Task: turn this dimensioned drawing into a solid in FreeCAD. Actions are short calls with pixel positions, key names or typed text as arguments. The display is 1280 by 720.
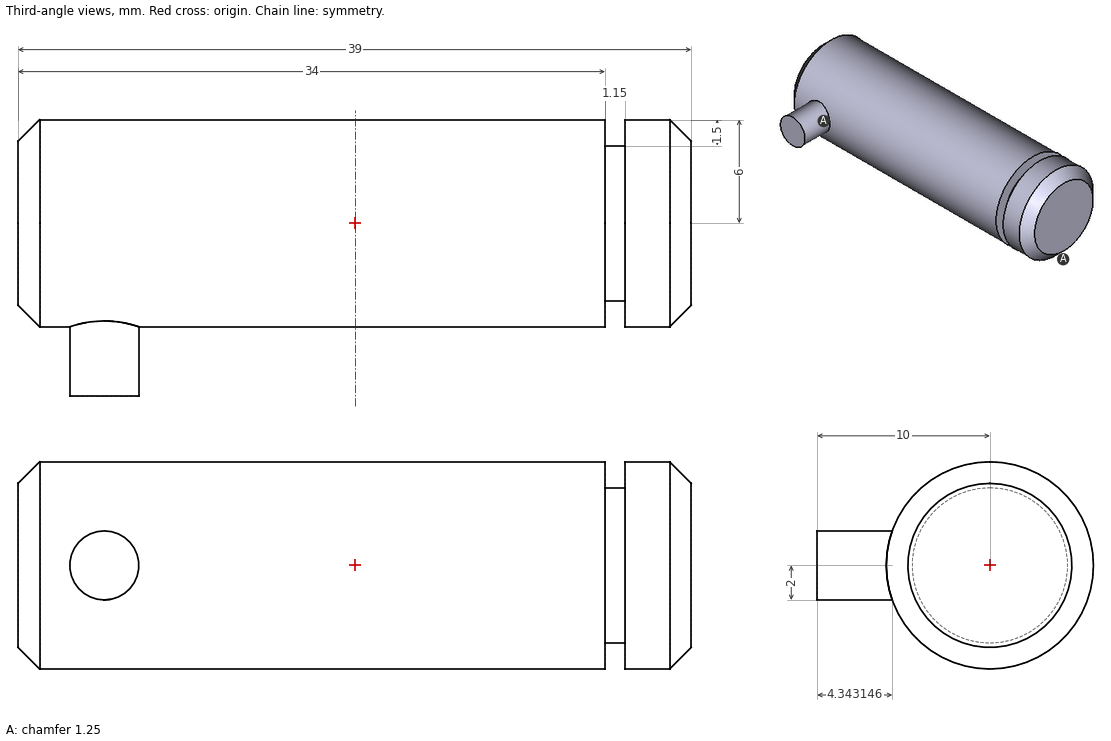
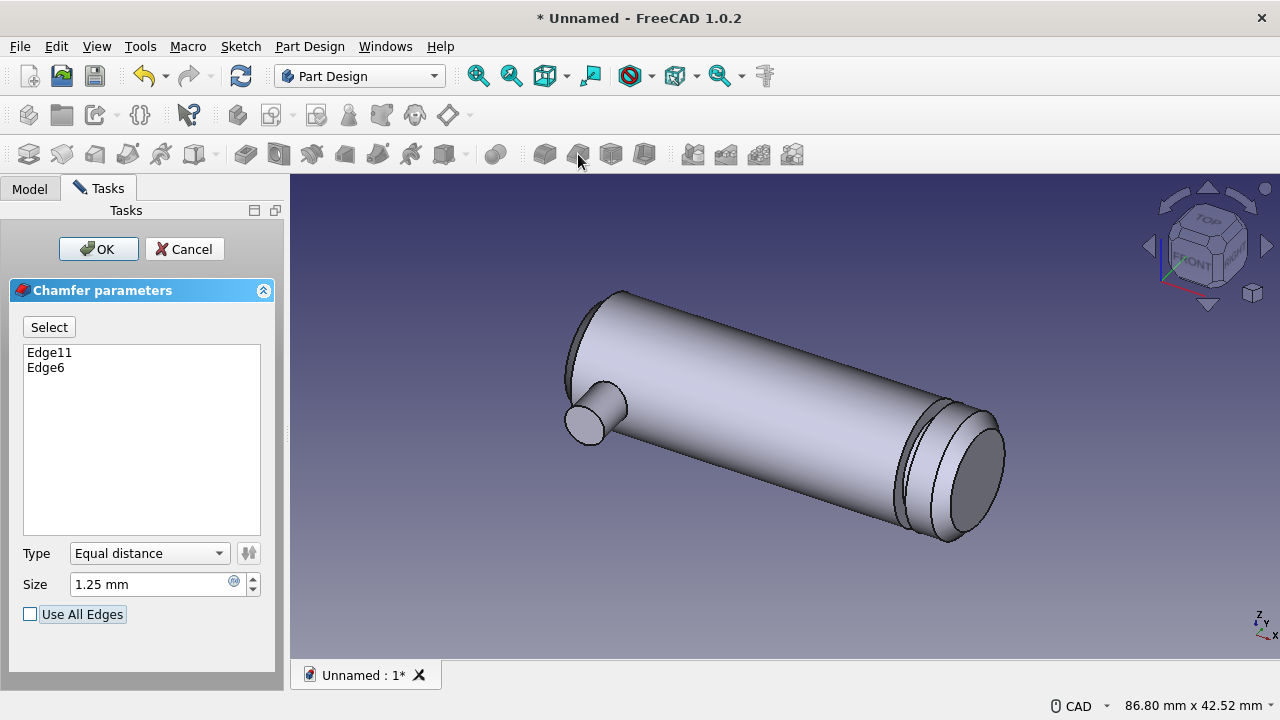
click(99, 249)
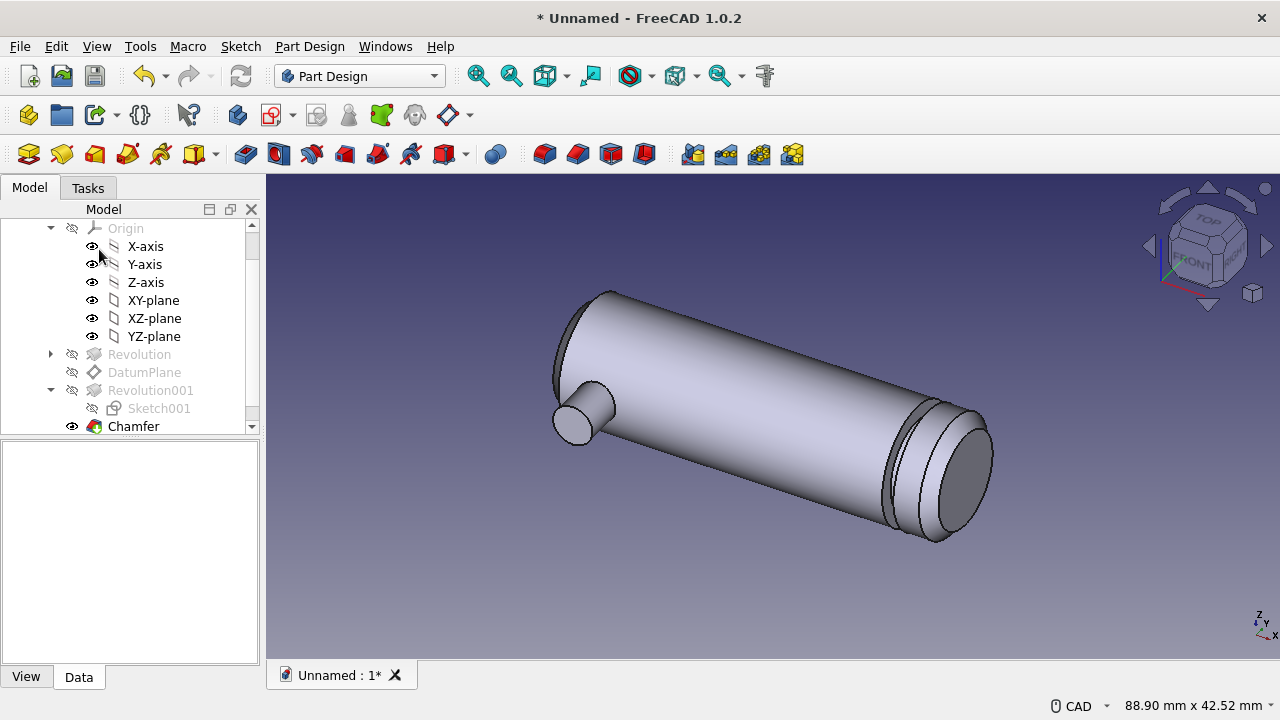
key(0)